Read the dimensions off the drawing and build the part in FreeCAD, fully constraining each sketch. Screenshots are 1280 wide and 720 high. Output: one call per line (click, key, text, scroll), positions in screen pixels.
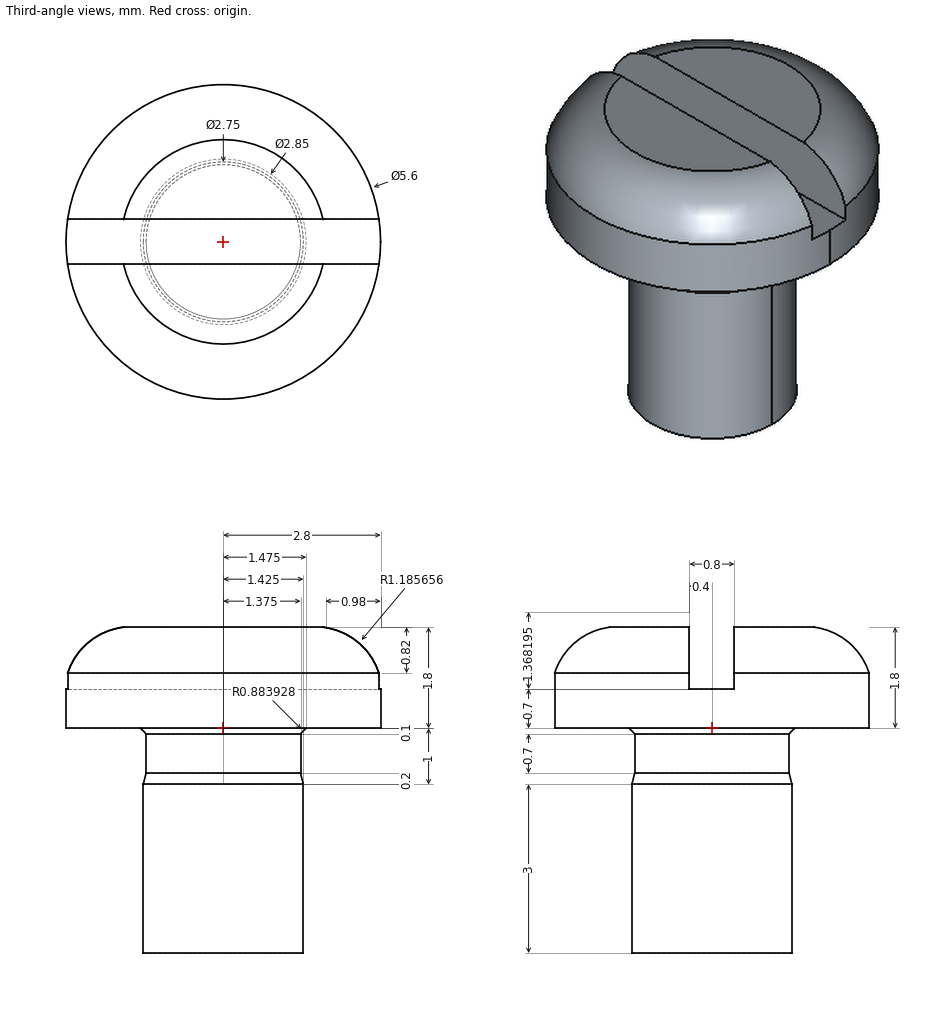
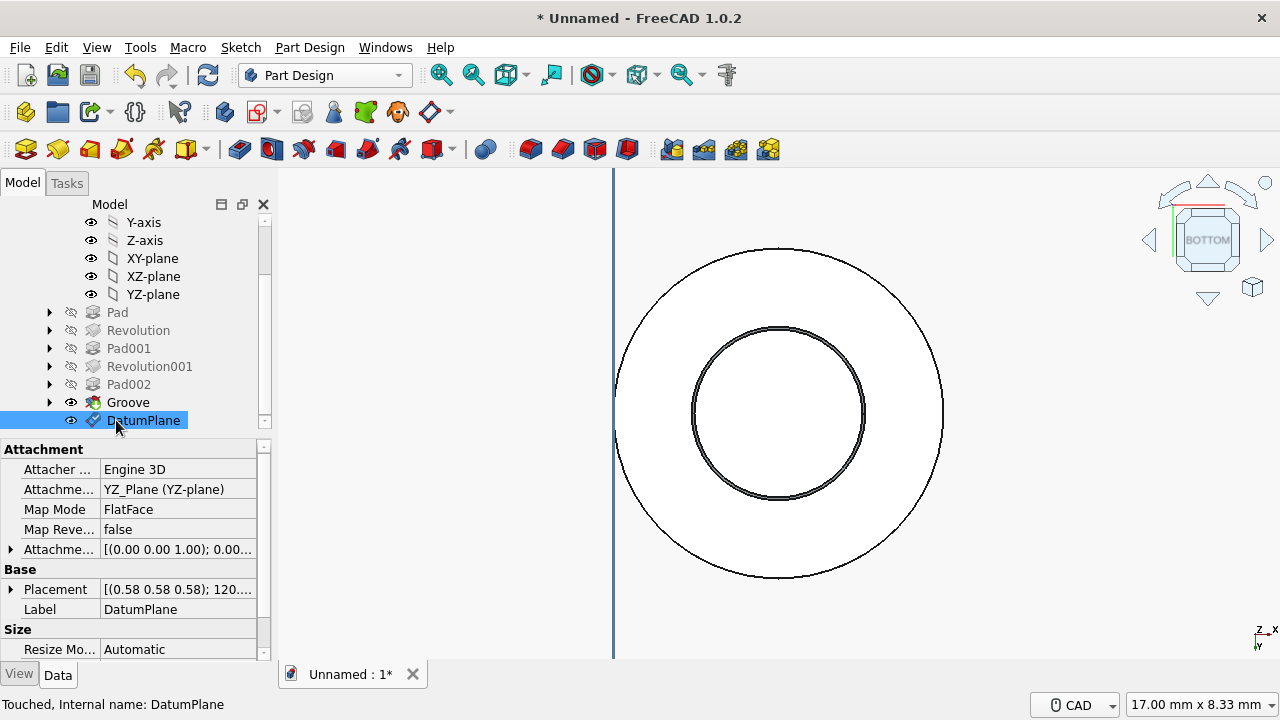
click(258, 112)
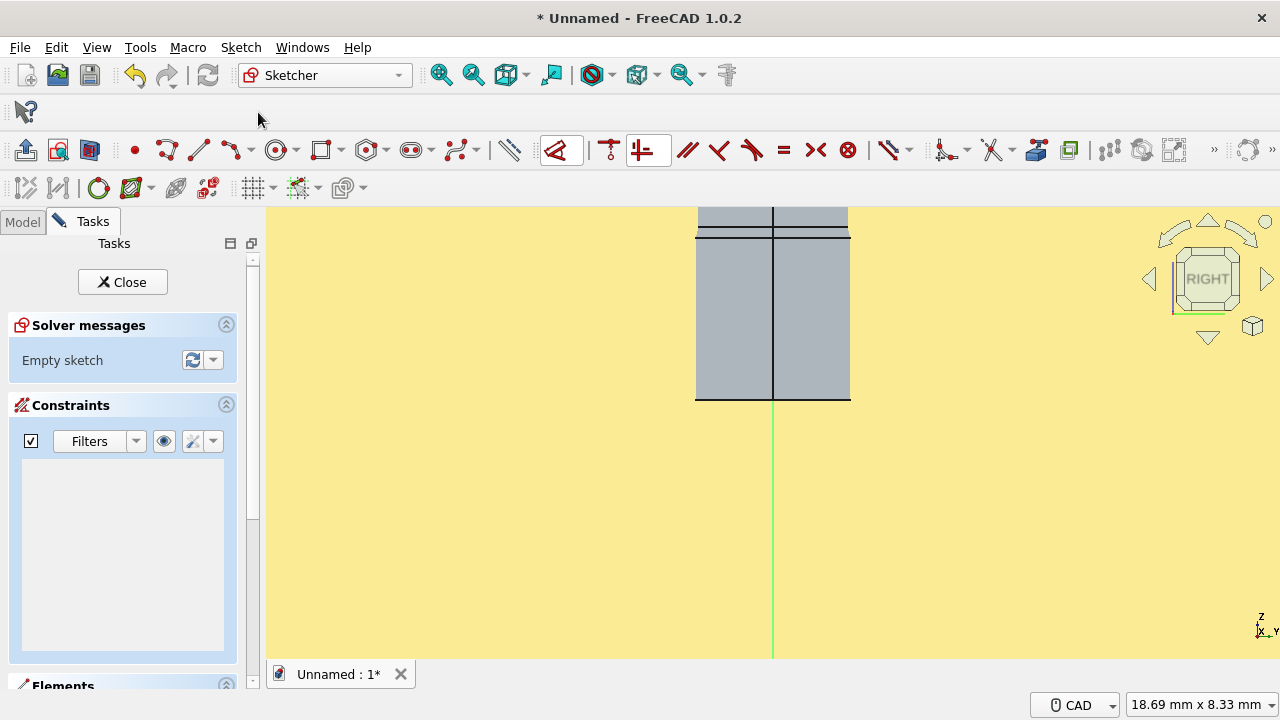
click(90, 150)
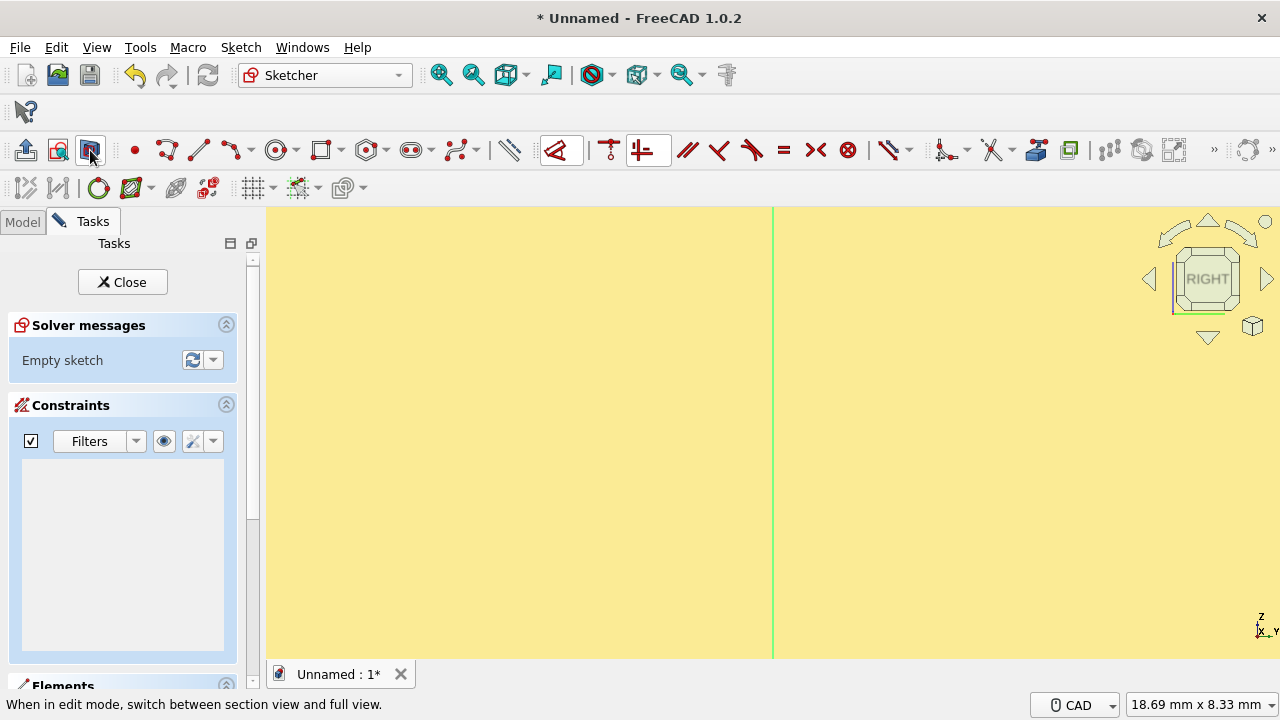
scroll(704, 433, down, 5)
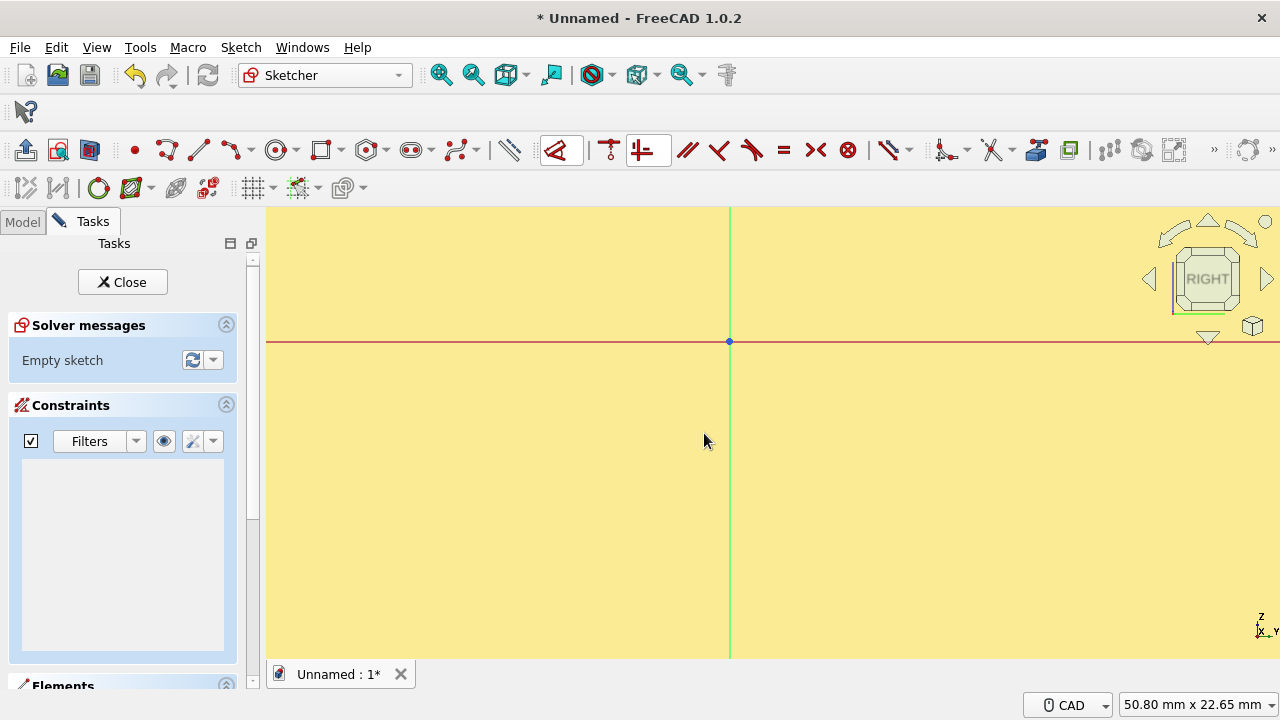
scroll(734, 303, up, 10)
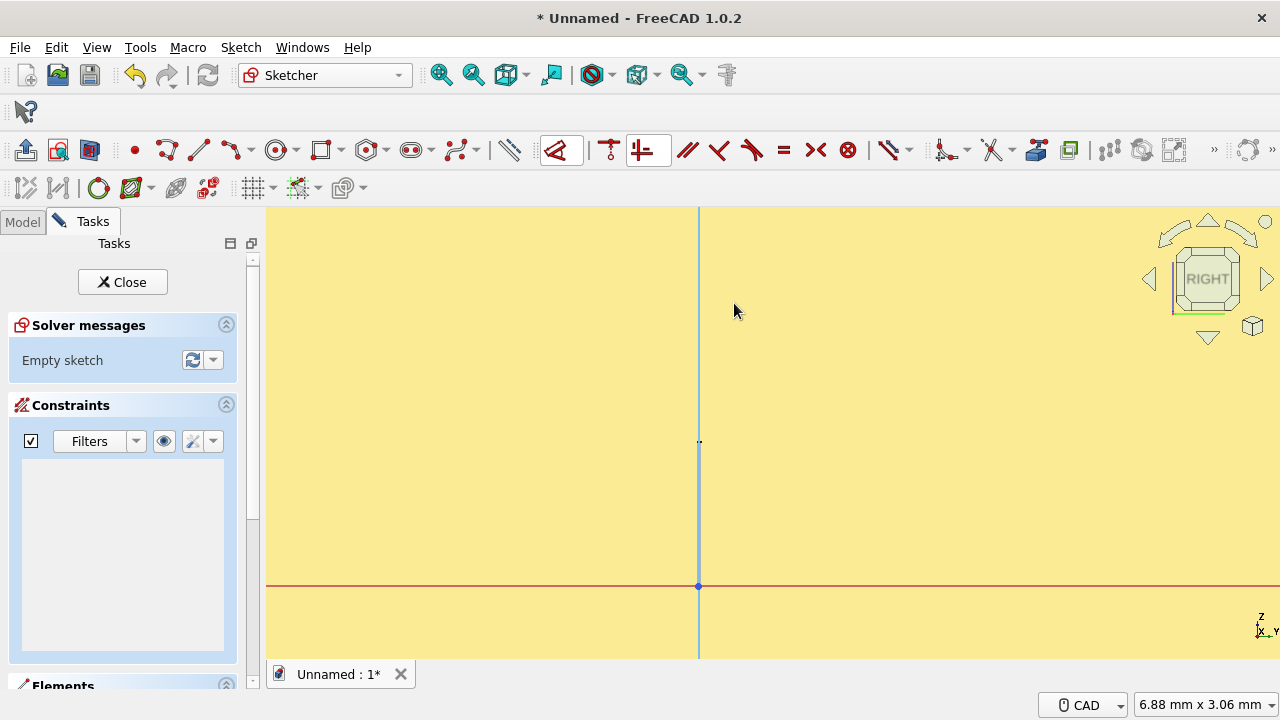
click(322, 150)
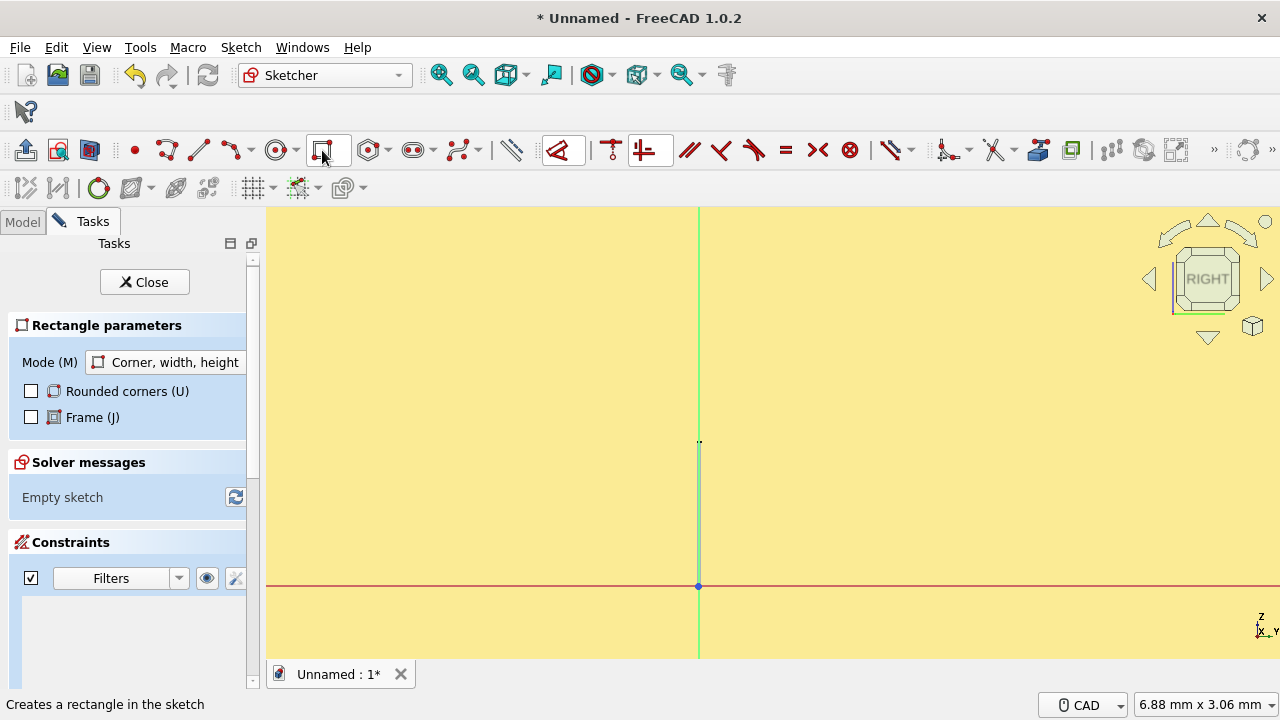
click(640, 281)
click(758, 483)
key(Escape)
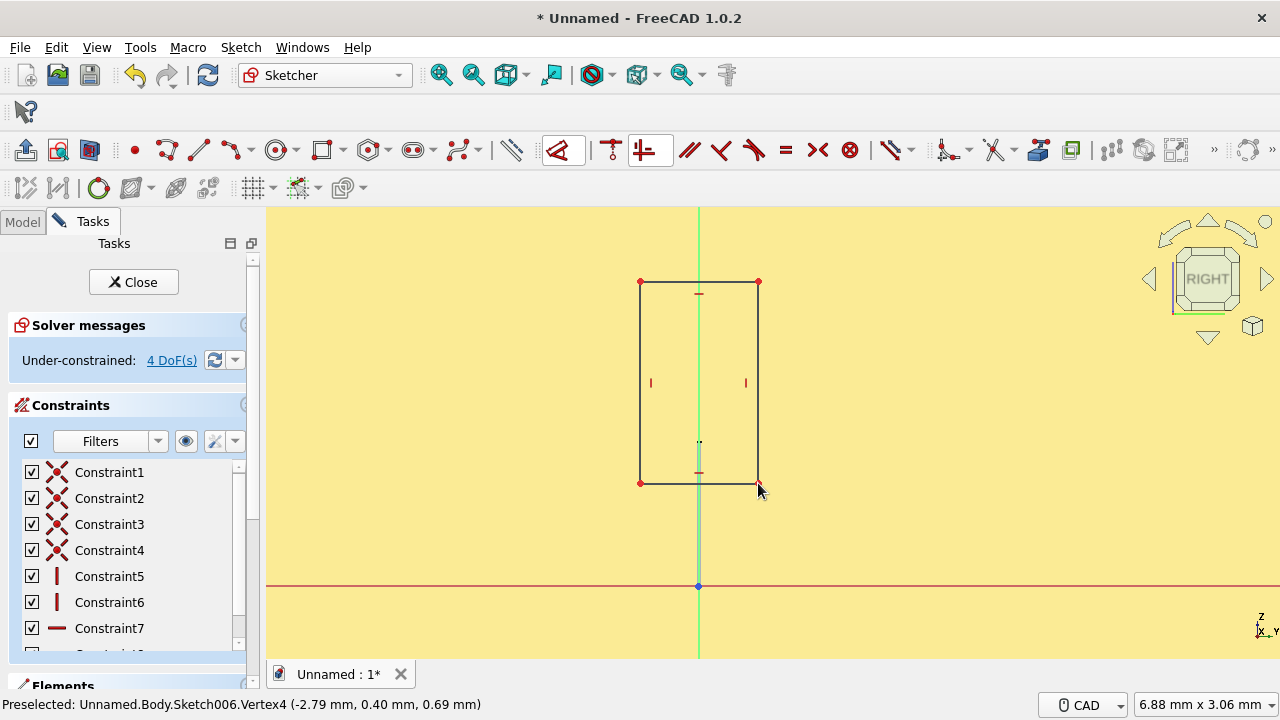
click(675, 484)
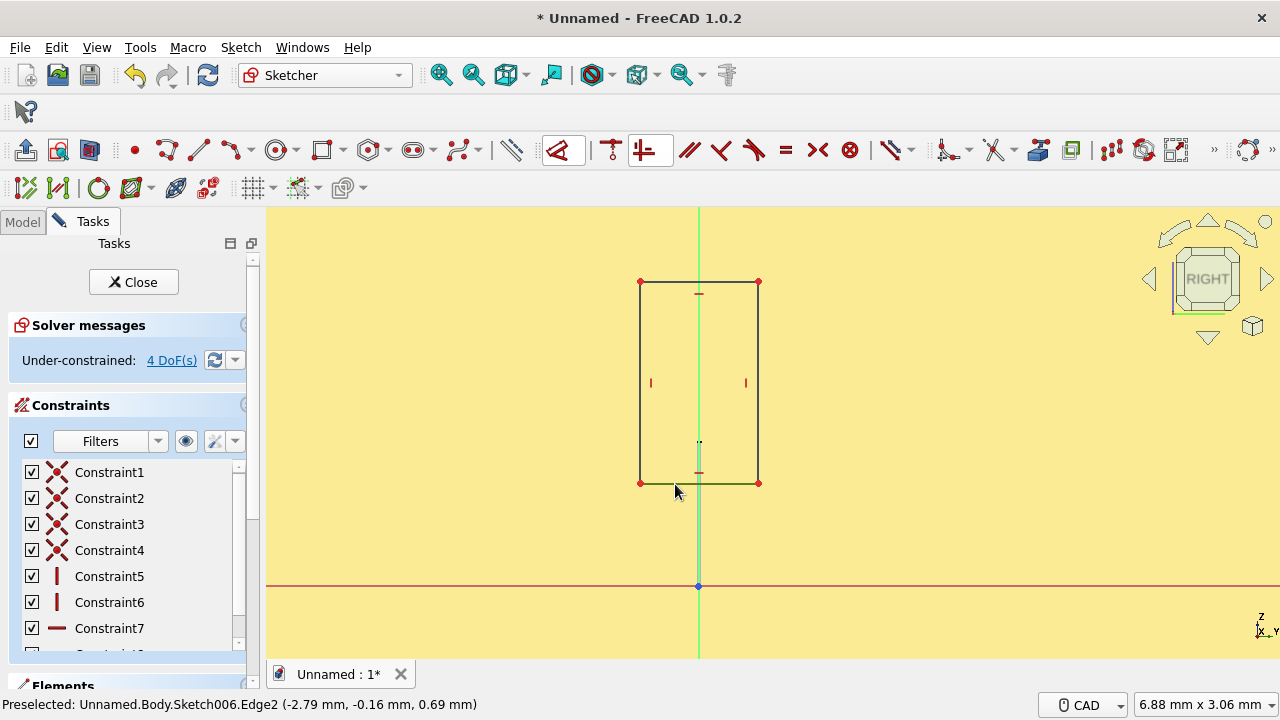
click(580, 150)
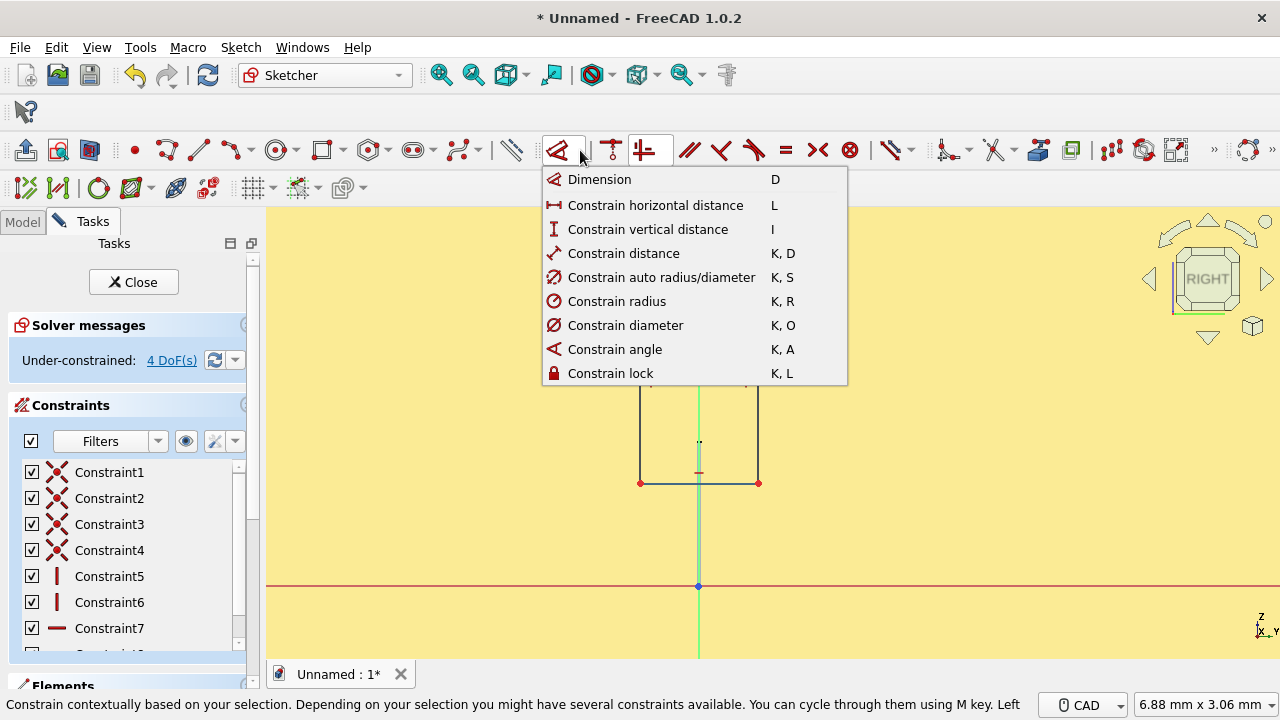
click(695, 205)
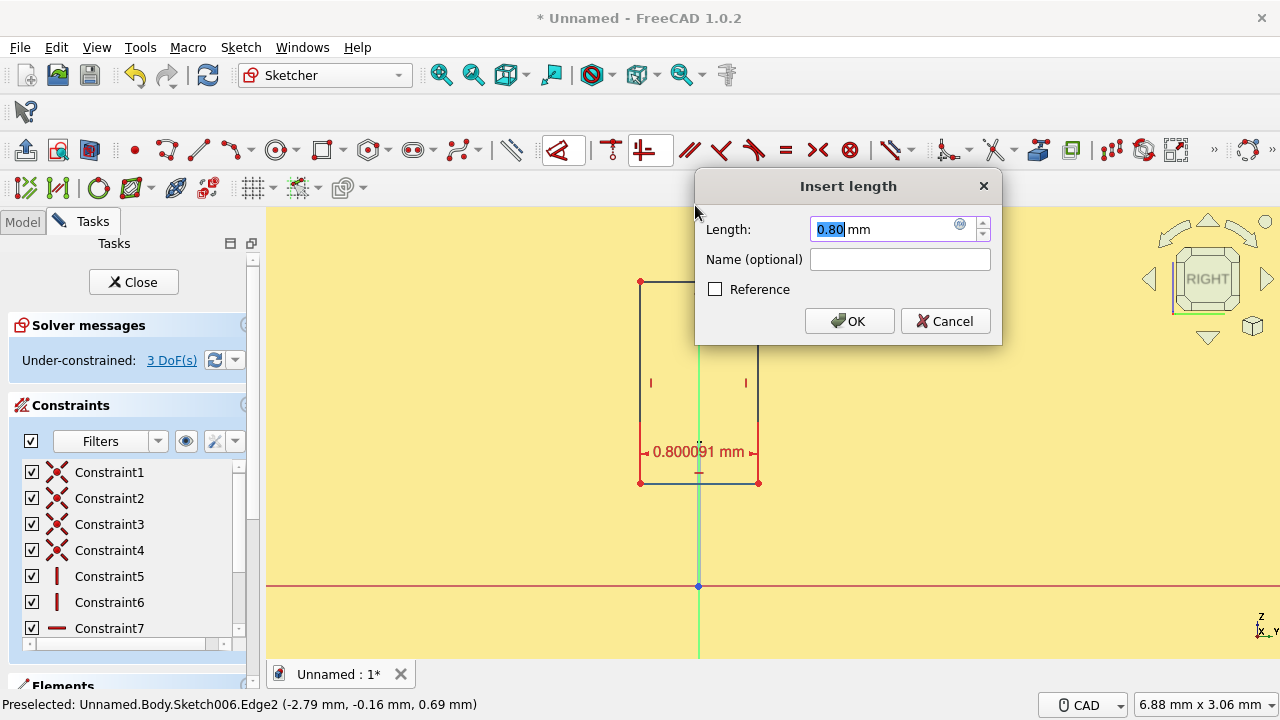
text(0.8)
key(Return)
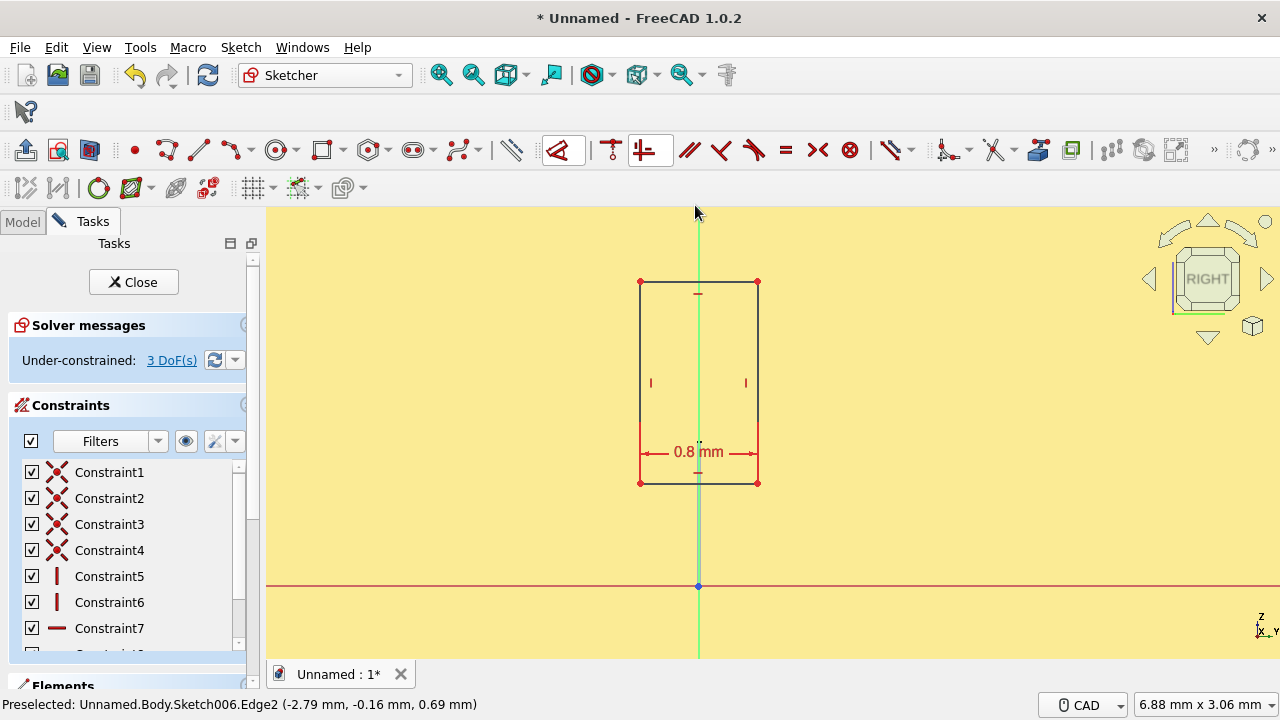
click(640, 282)